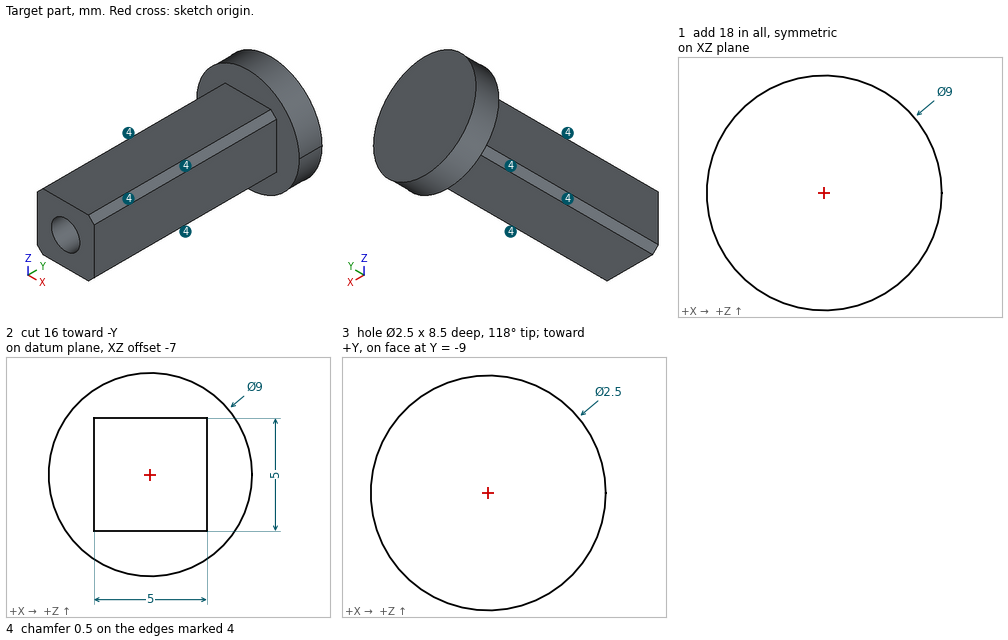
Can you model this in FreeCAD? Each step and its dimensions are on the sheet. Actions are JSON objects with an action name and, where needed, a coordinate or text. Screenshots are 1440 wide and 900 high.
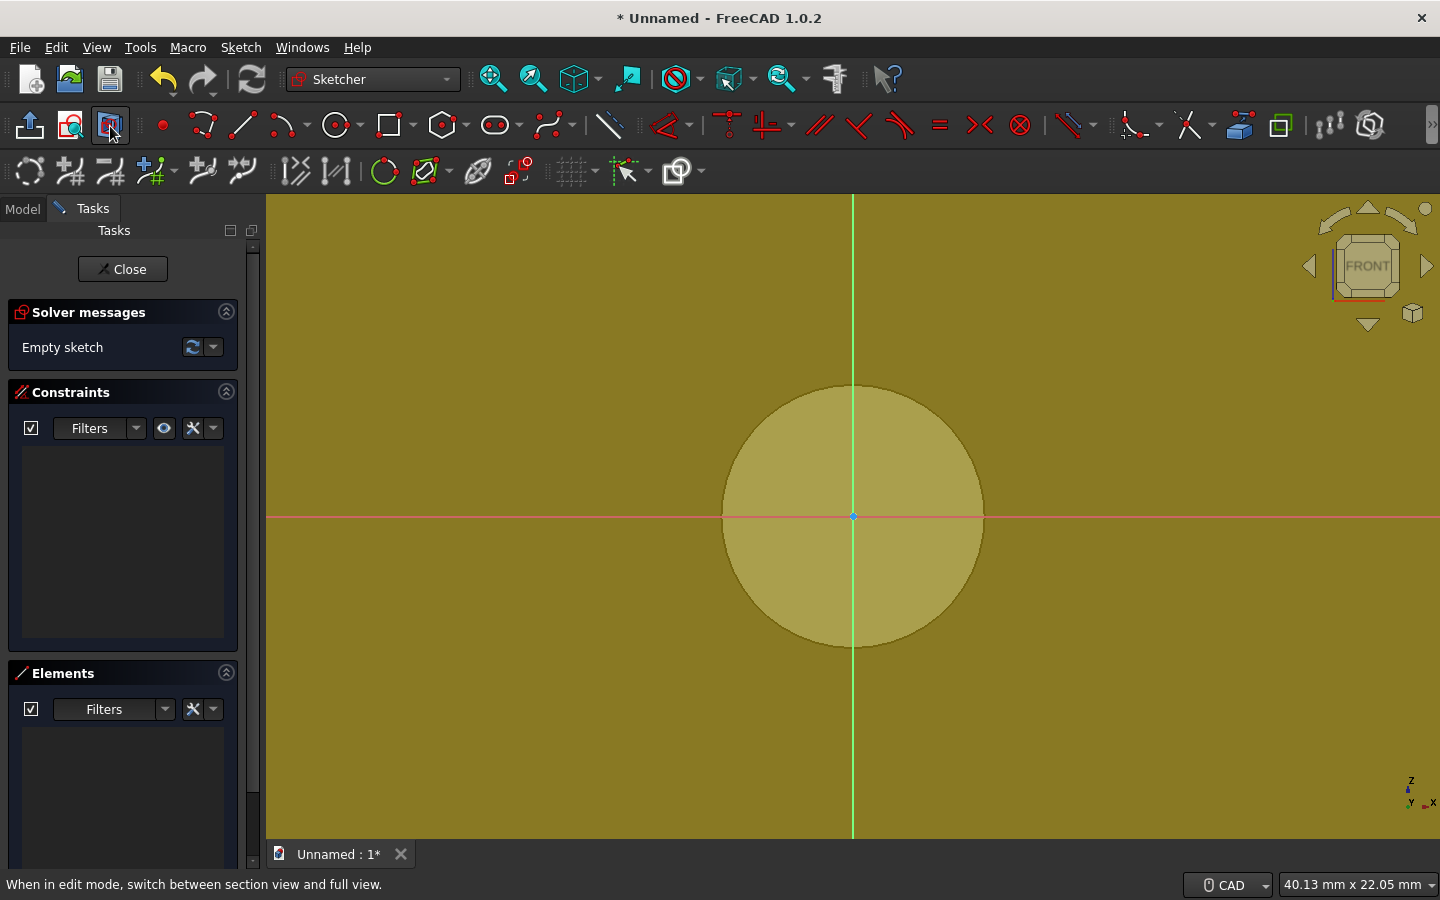
{"action": "scroll", "coordinate": [992, 517], "scroll_direction": "up", "scroll_amount": 2}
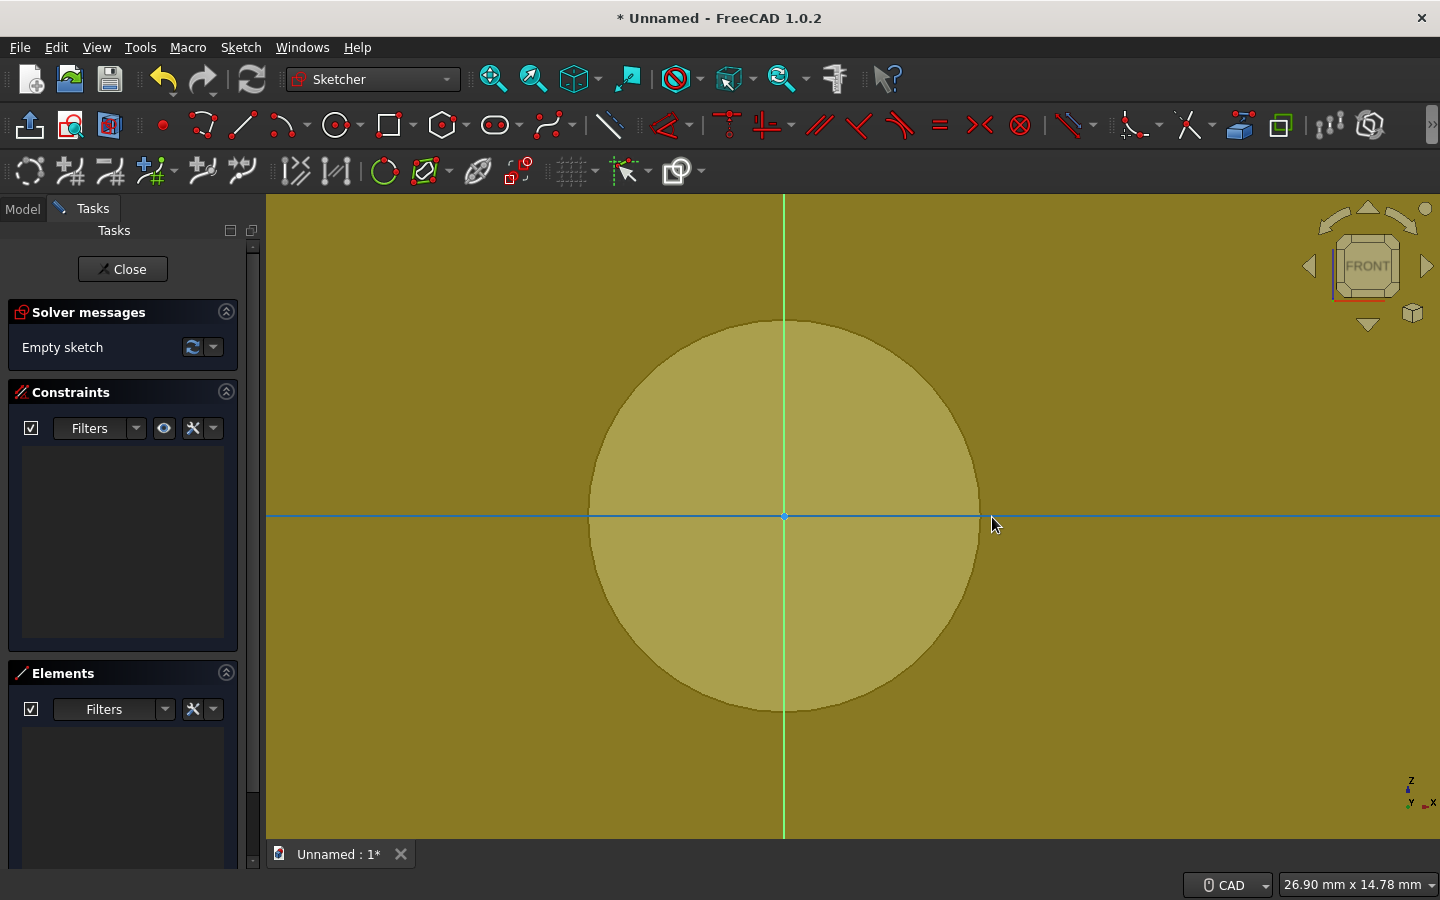
{"action": "left_click", "coordinate": [416, 126]}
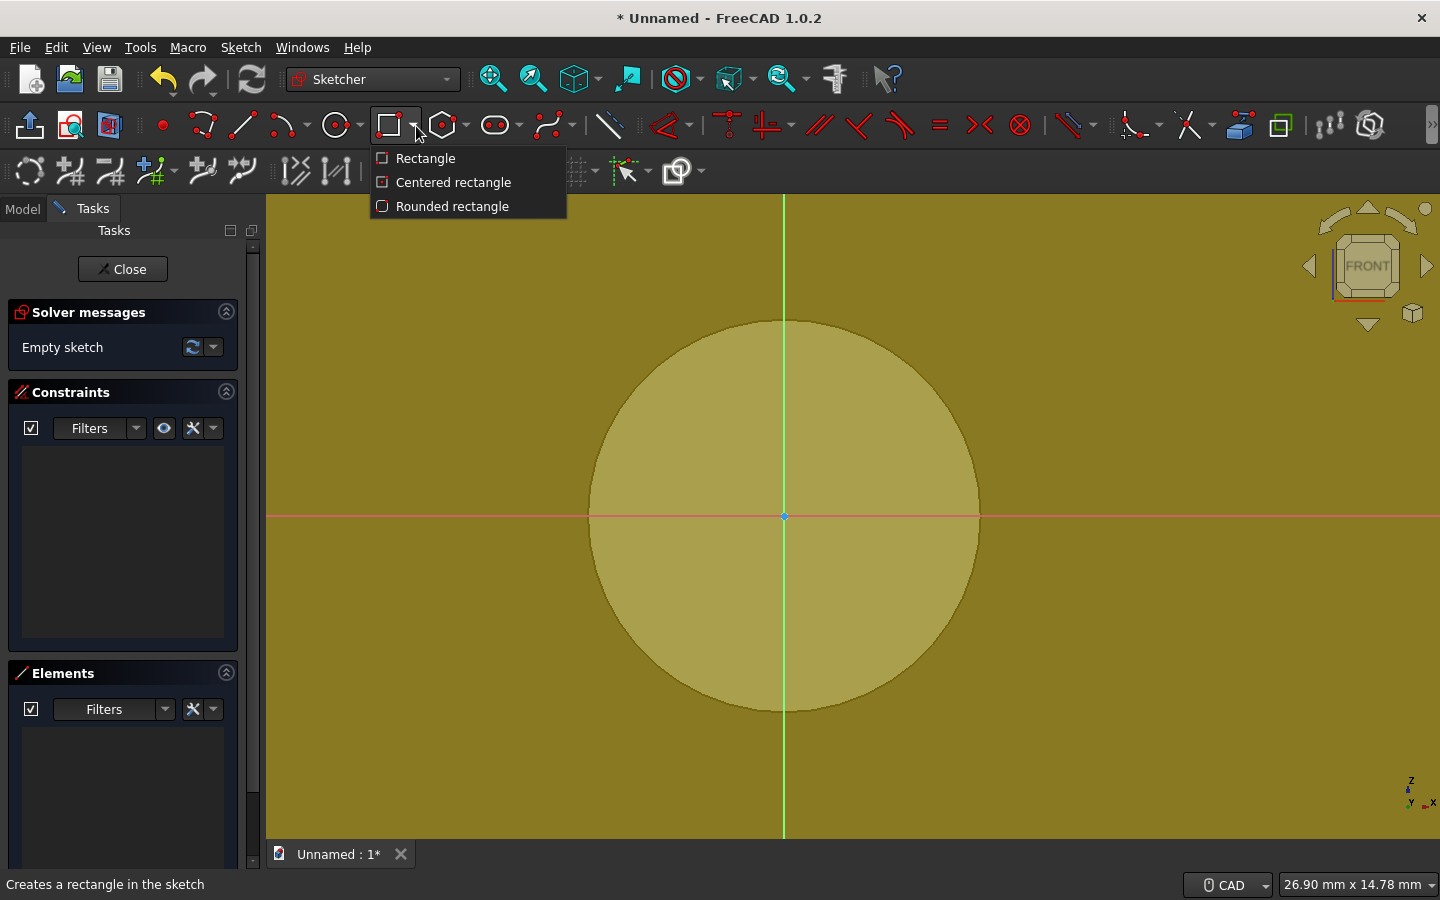
{"action": "left_click", "coordinate": [468, 182]}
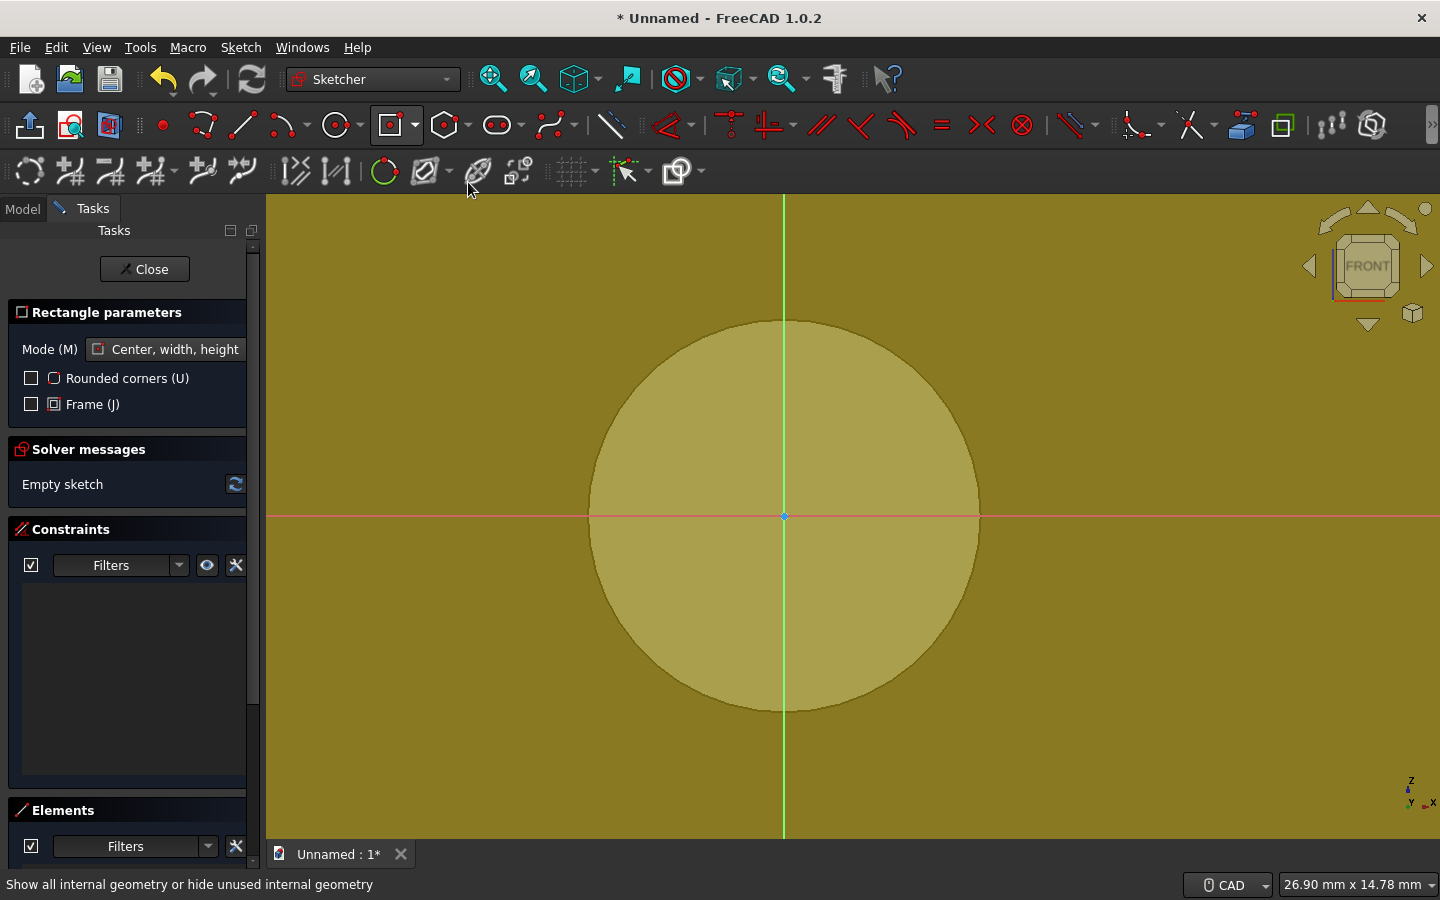
{"action": "left_click", "coordinate": [784, 516]}
{"action": "mouse_move", "coordinate": [893, 407]}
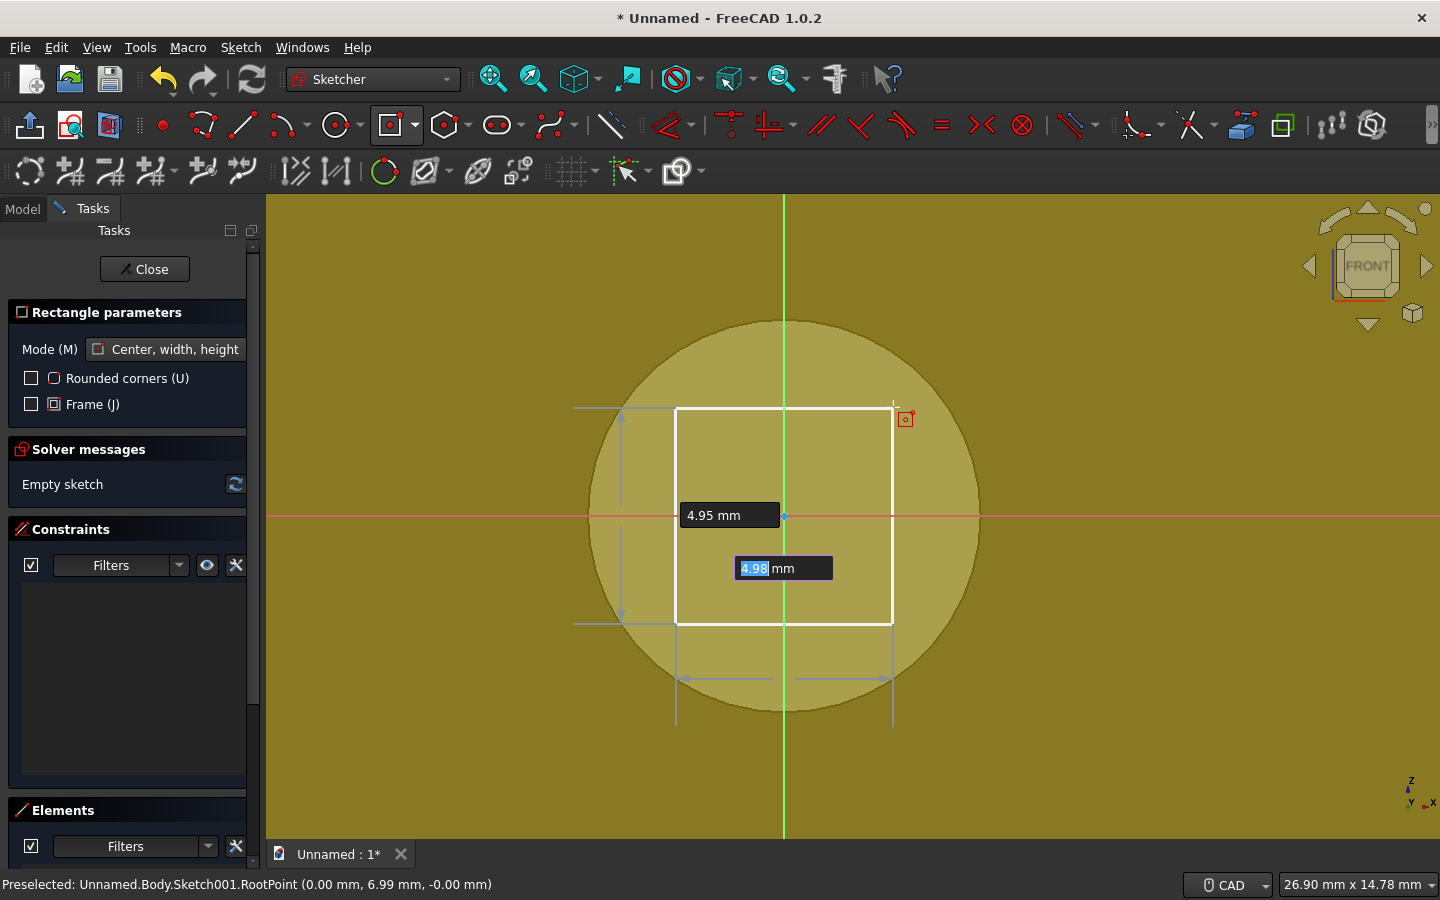
{"action": "type", "text": "5"}
{"action": "key", "text": "Tab"}
{"action": "type", "text": "5"}
{"action": "key", "text": "Return"}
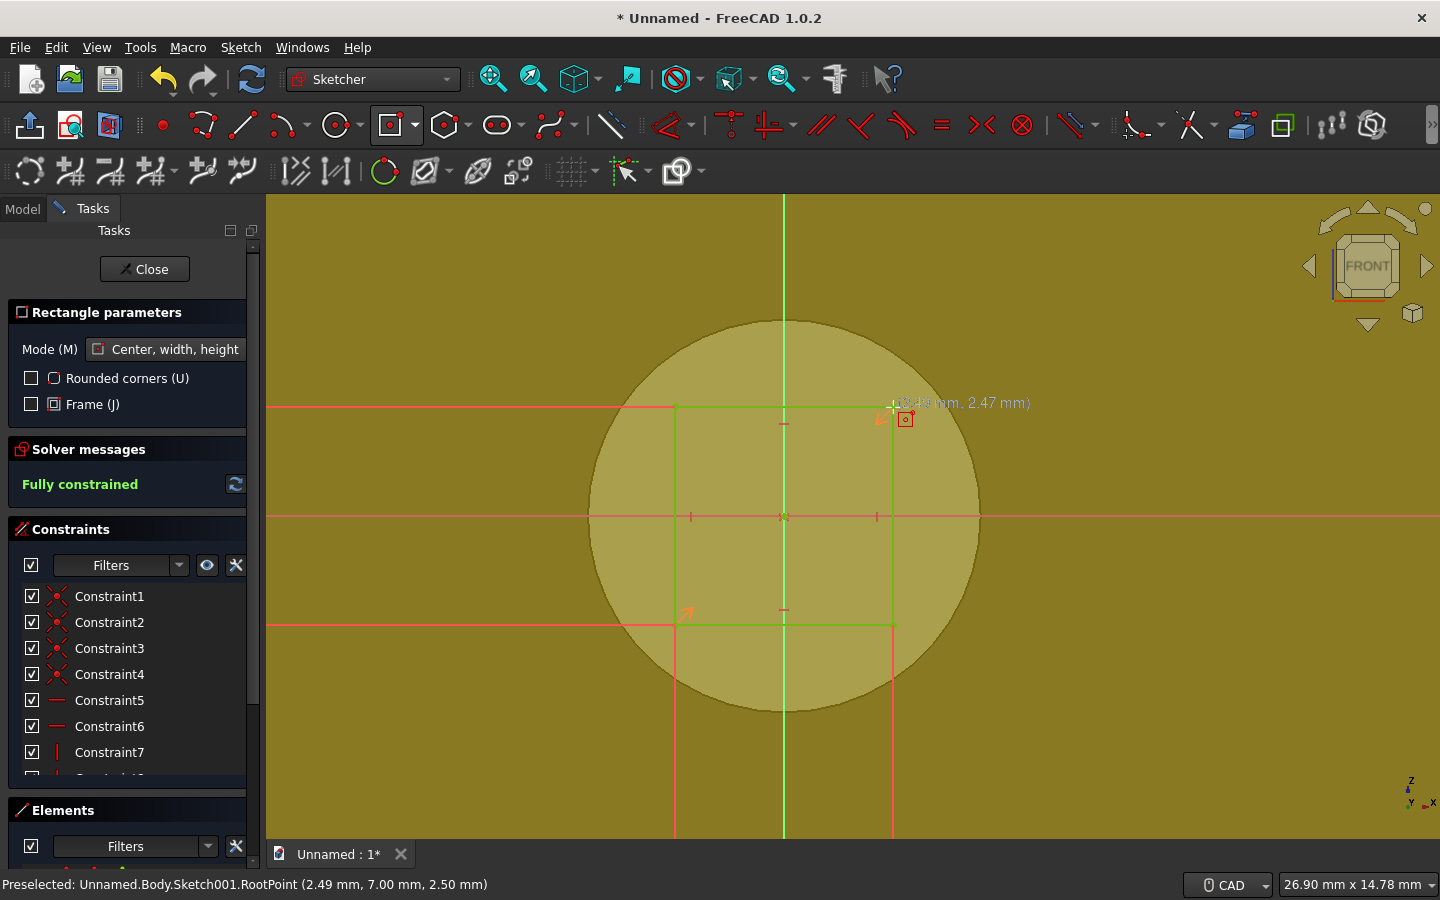
{"action": "left_click", "coordinate": [336, 126]}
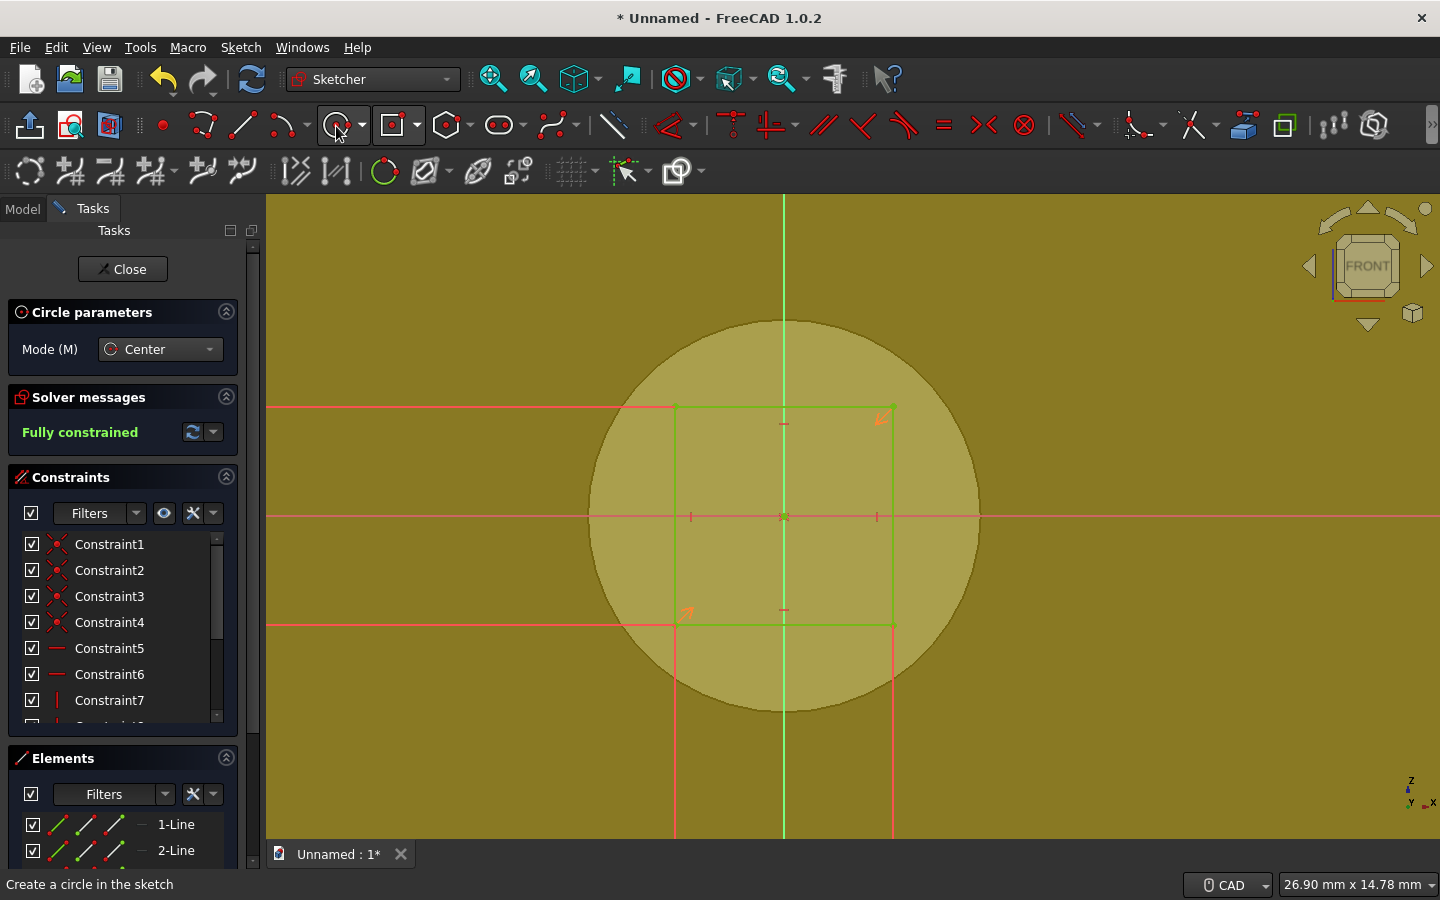
{"action": "left_click", "coordinate": [784, 516]}
{"action": "mouse_move", "coordinate": [923, 377]}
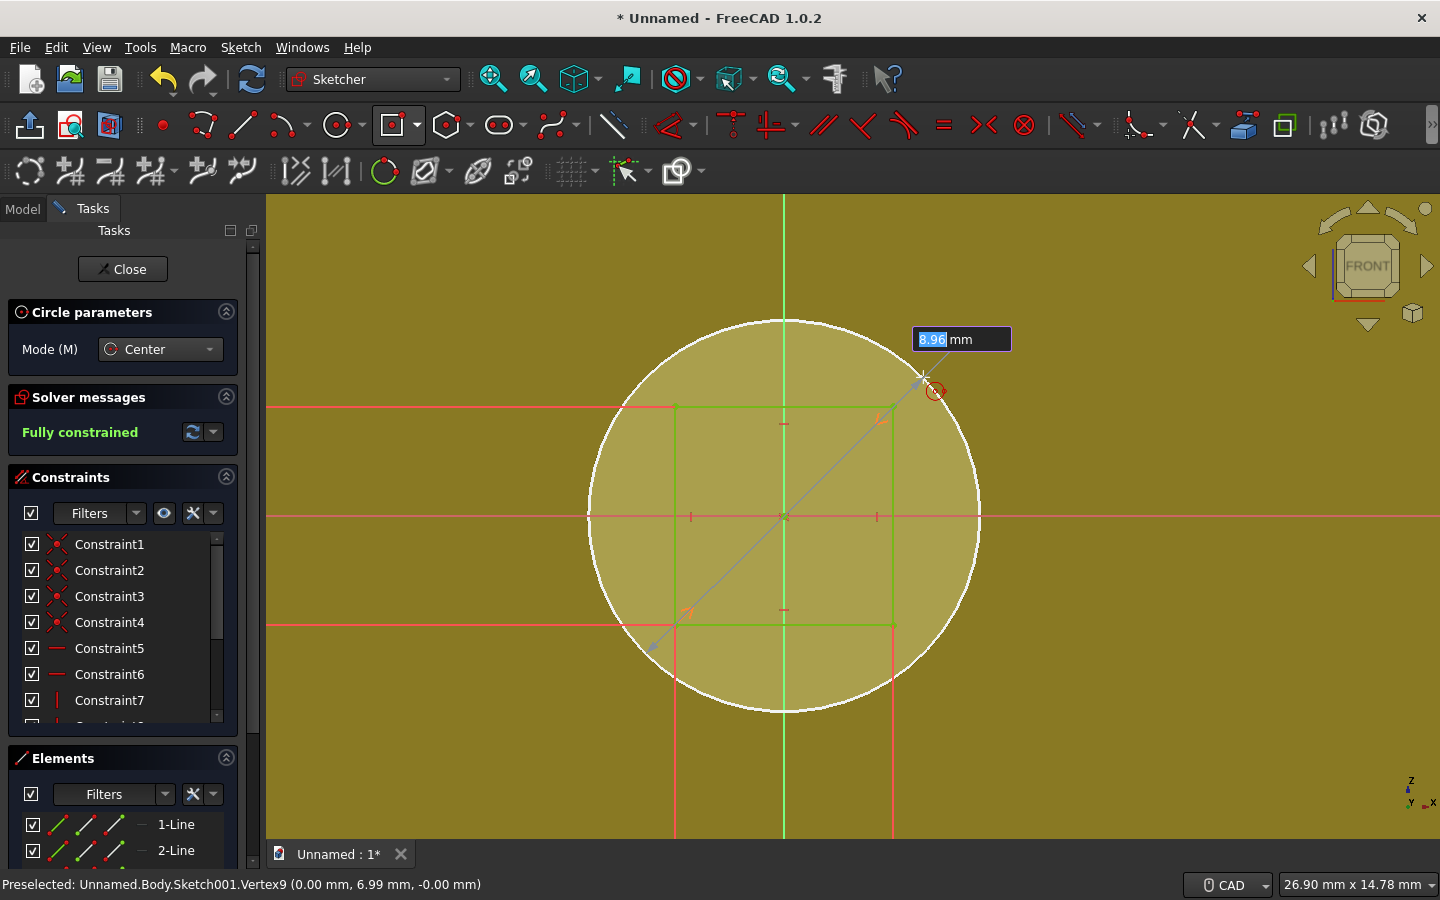
{"action": "type", "text": "9"}
{"action": "key", "text": "Return"}
{"action": "key", "text": "Escape"}